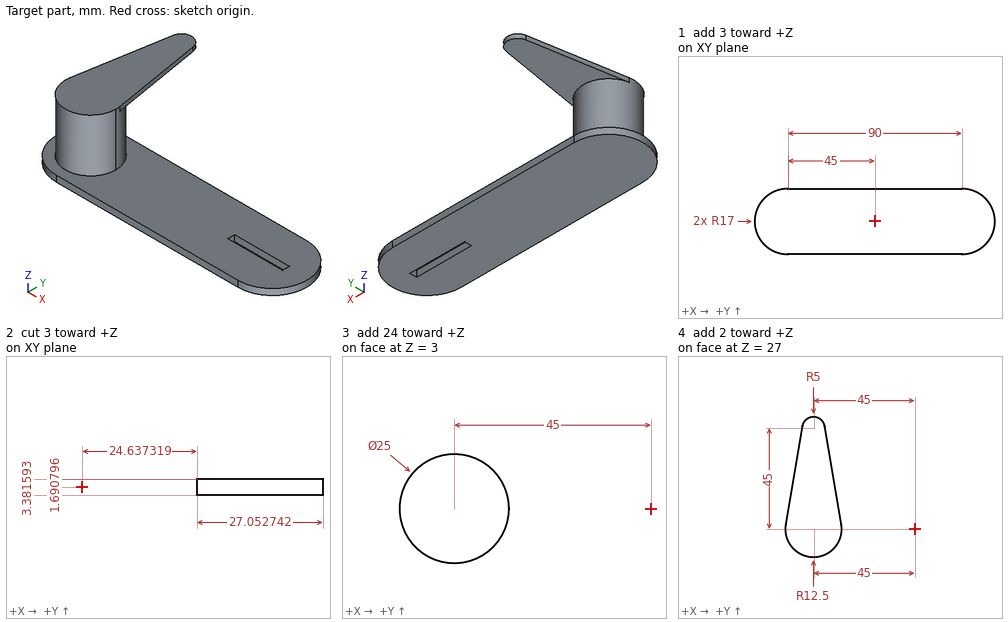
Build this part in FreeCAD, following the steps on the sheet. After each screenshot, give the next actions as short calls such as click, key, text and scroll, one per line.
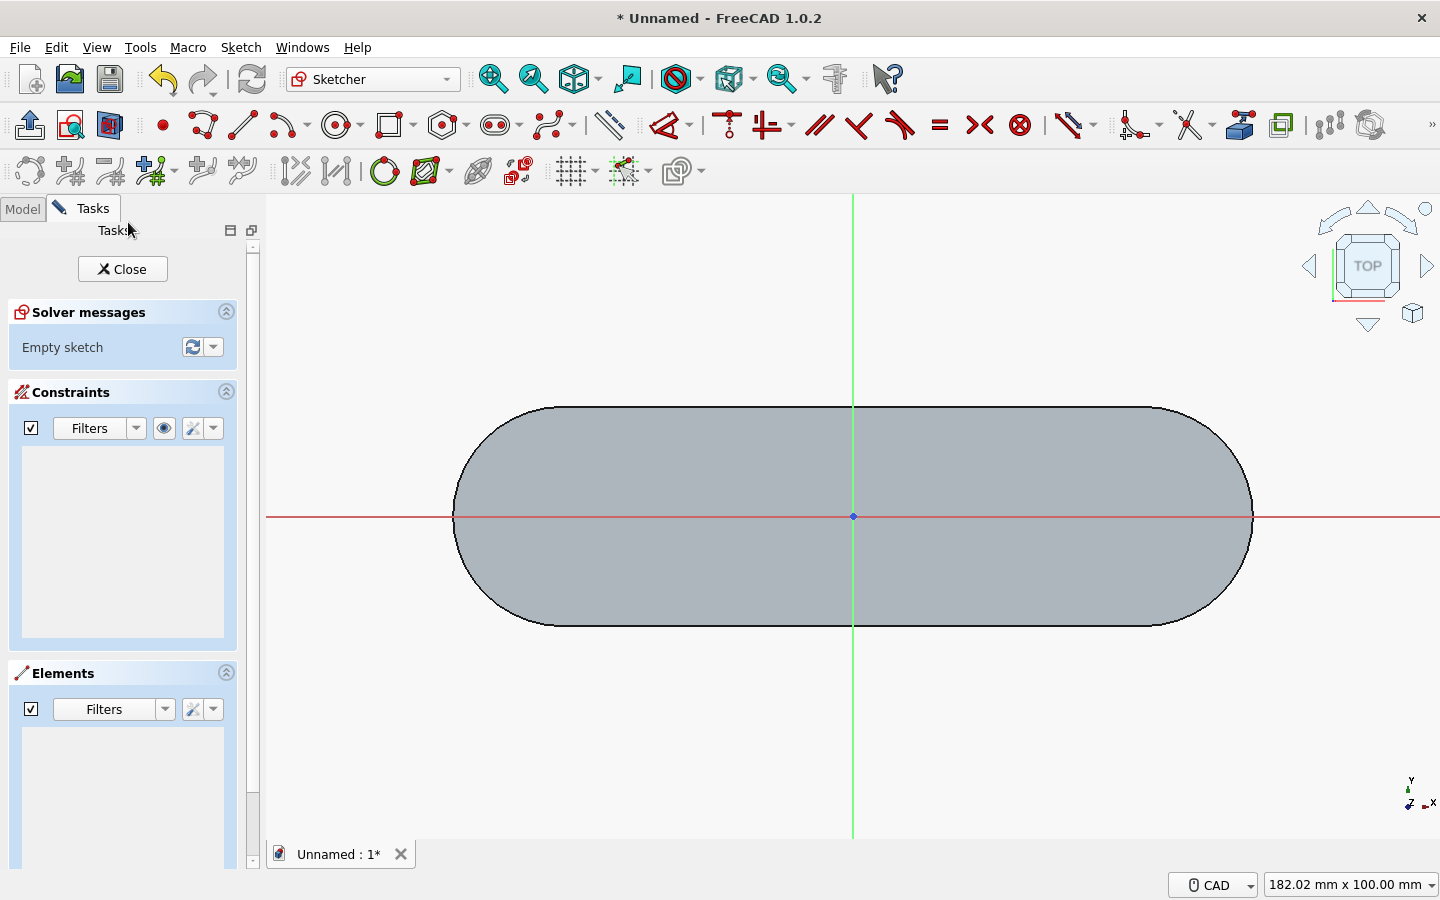
scroll(1212, 517, up, 4)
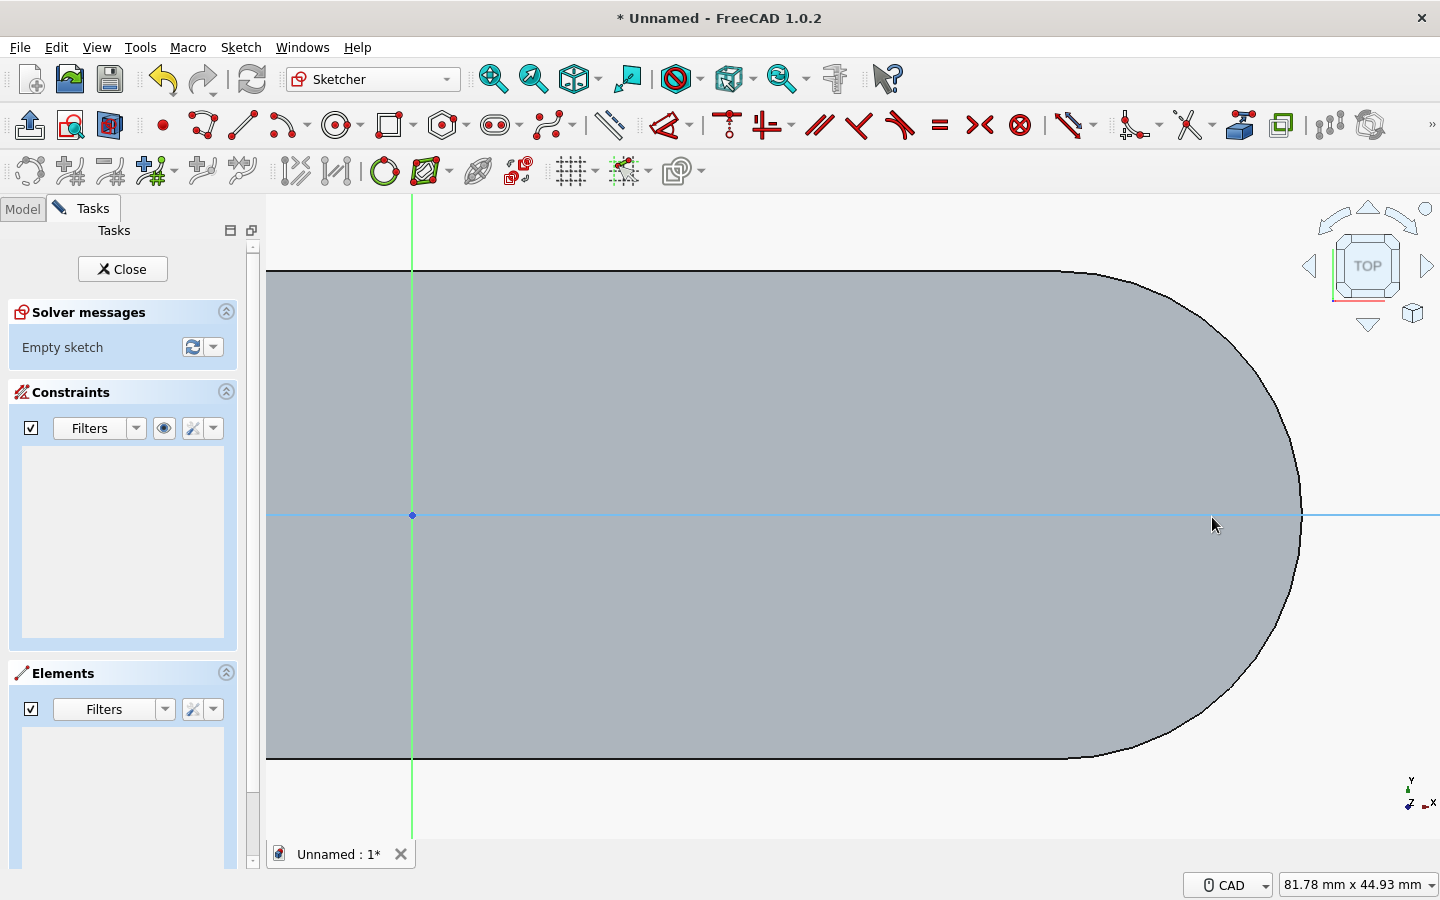
click(390, 126)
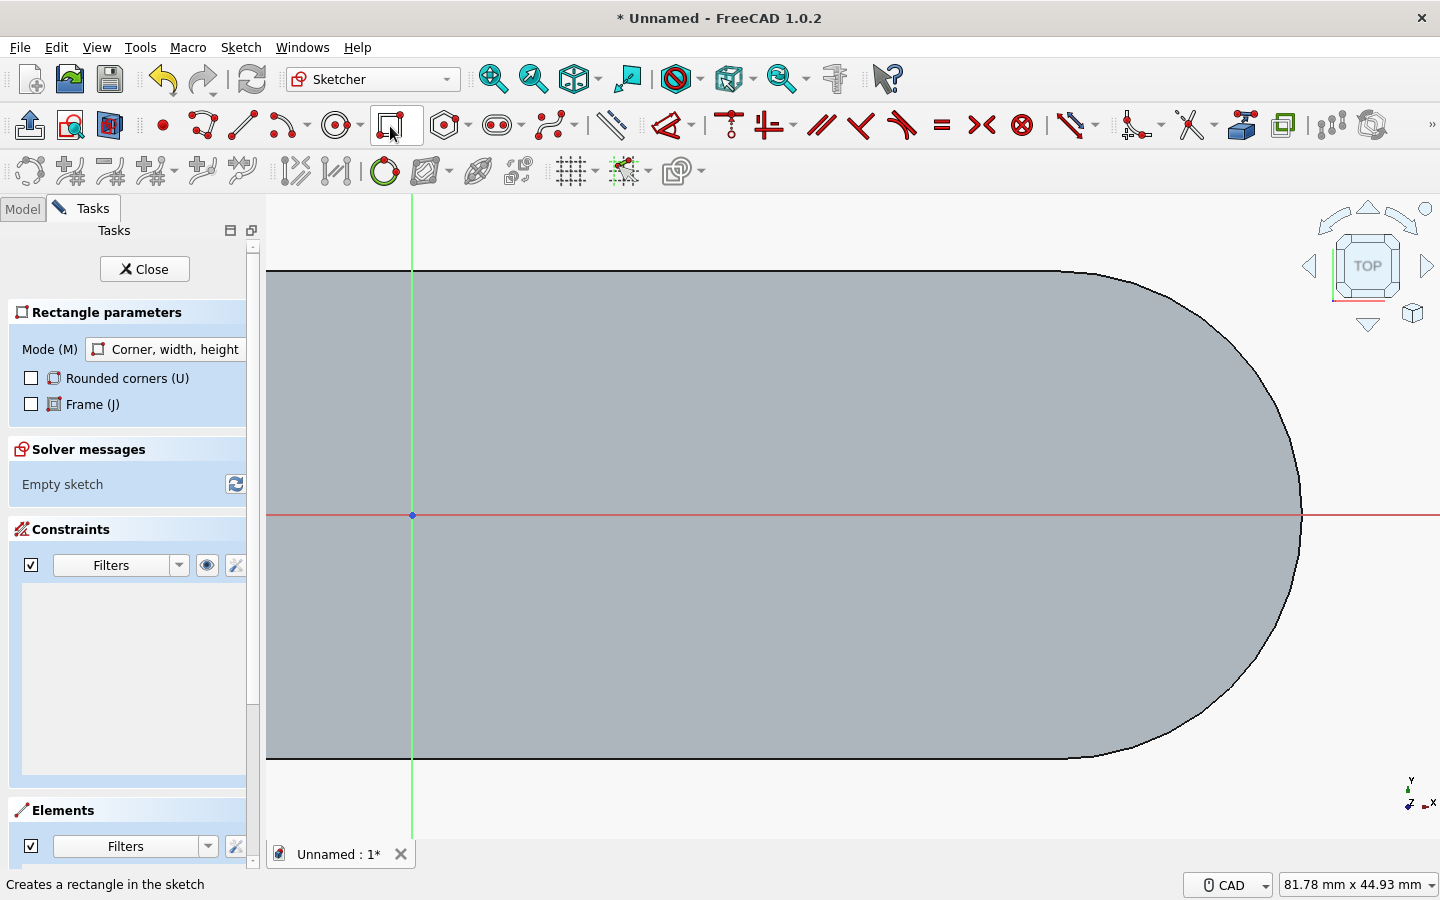
click(766, 491)
click(1154, 540)
key(Escape)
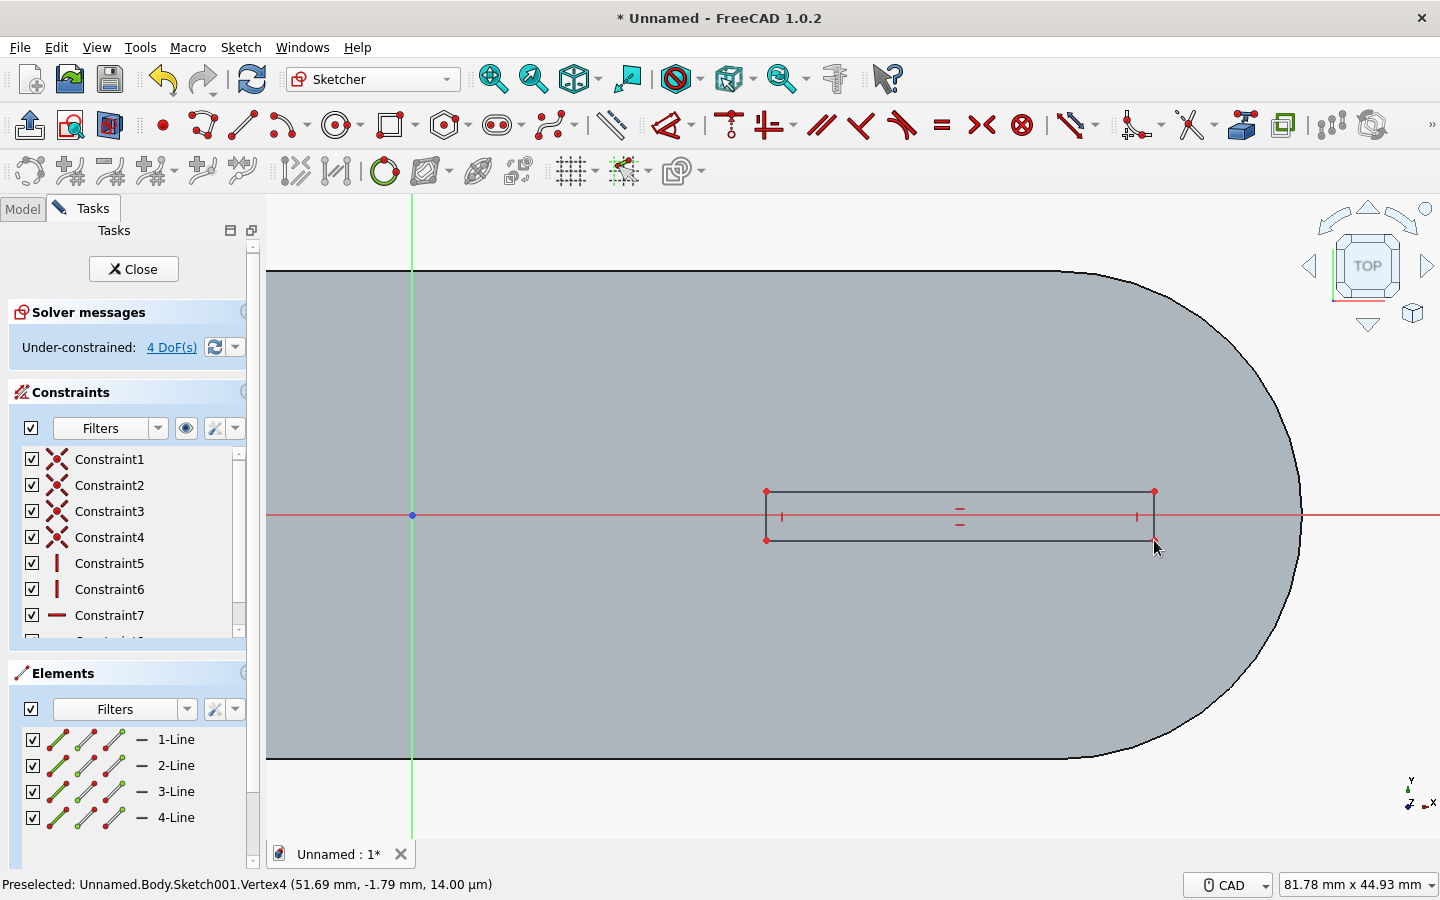
key(d)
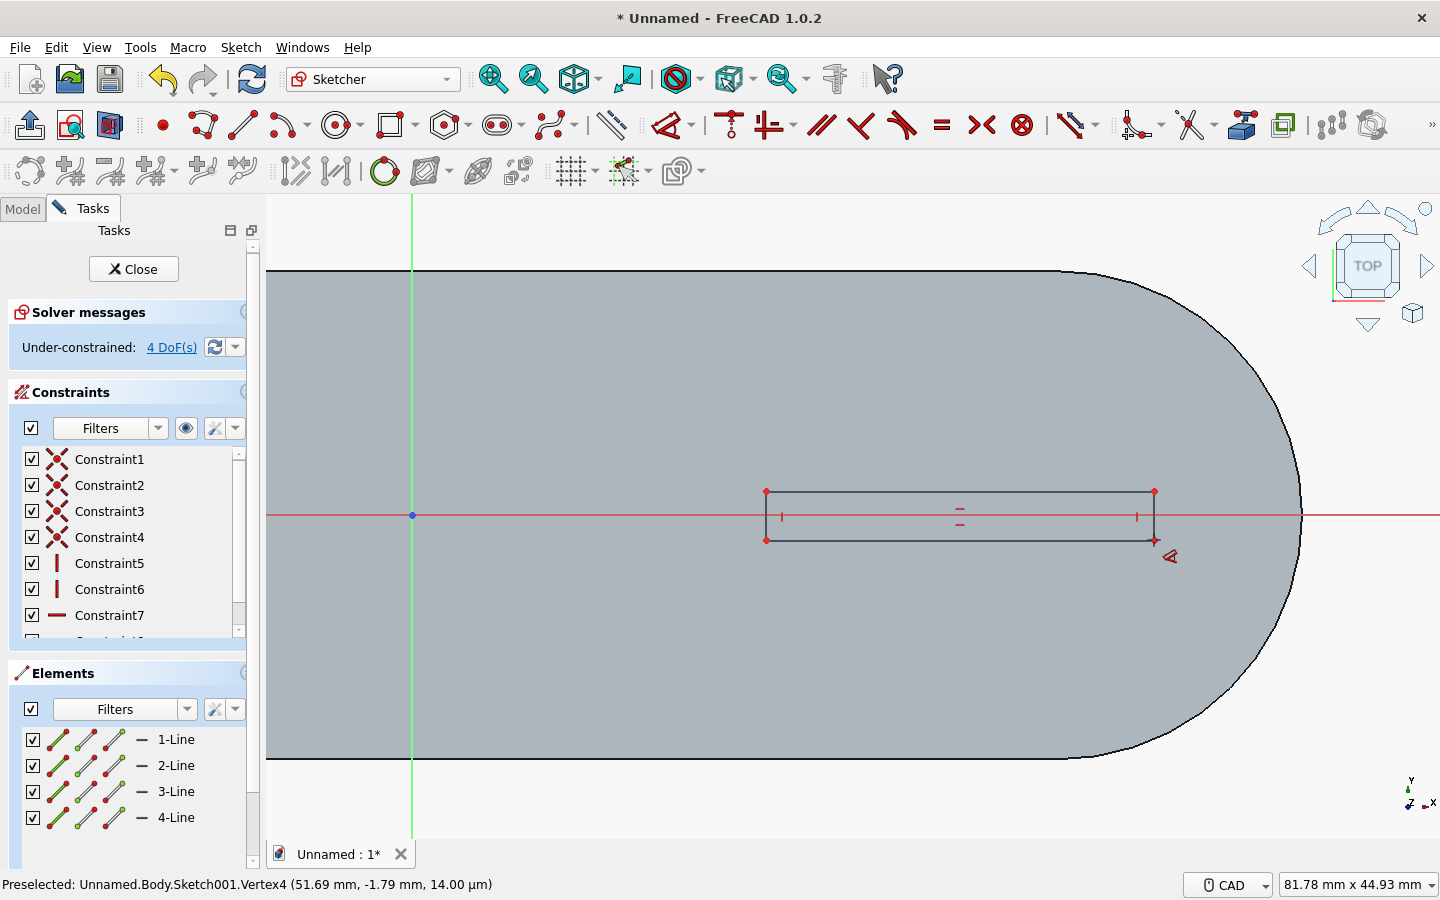
scroll(766, 526, up, 2)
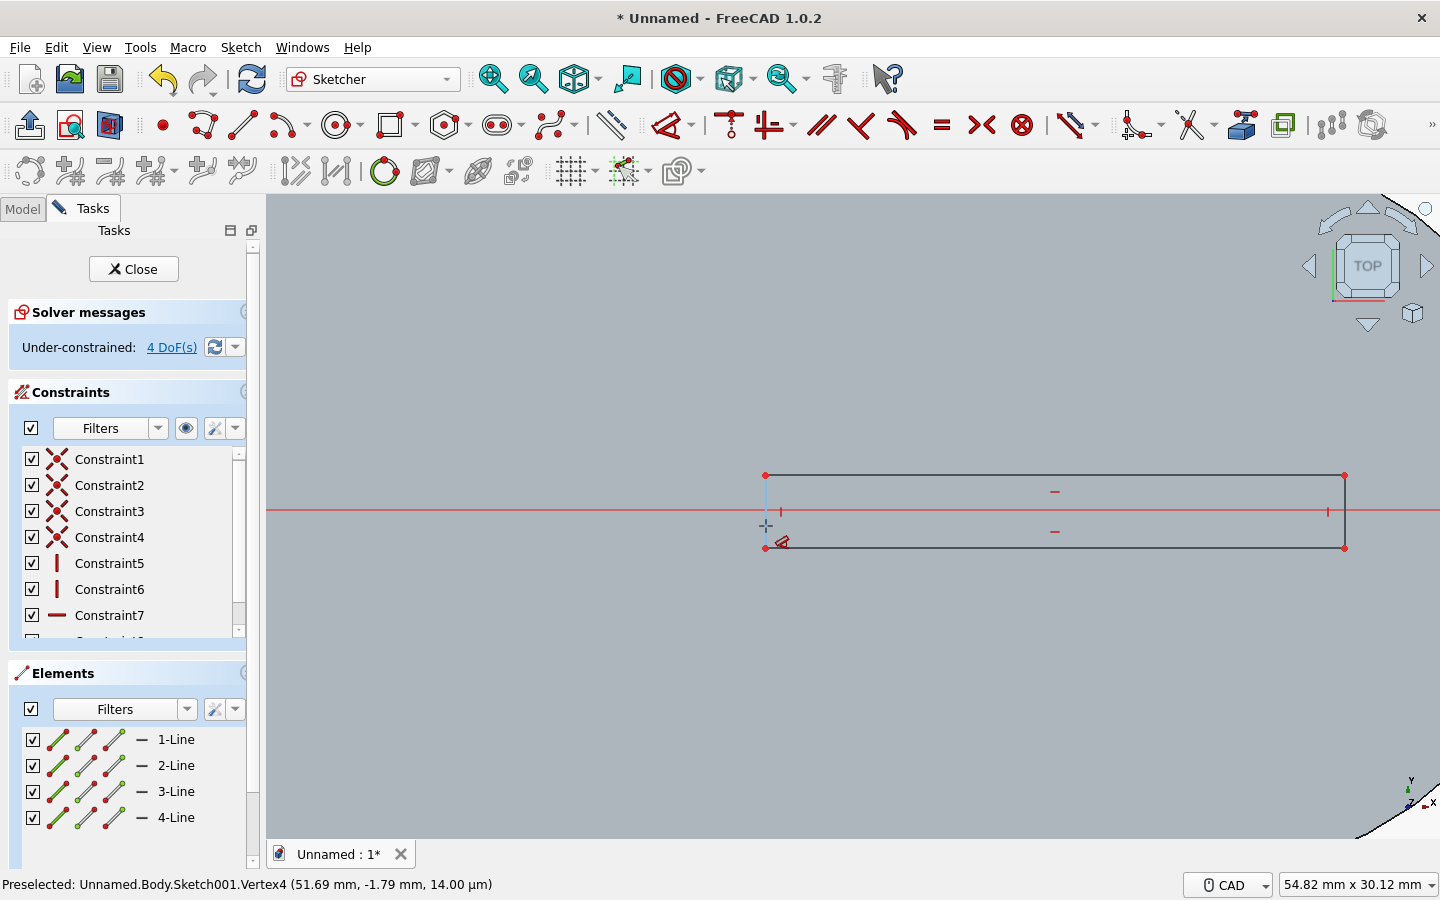
click(766, 526)
click(732, 495)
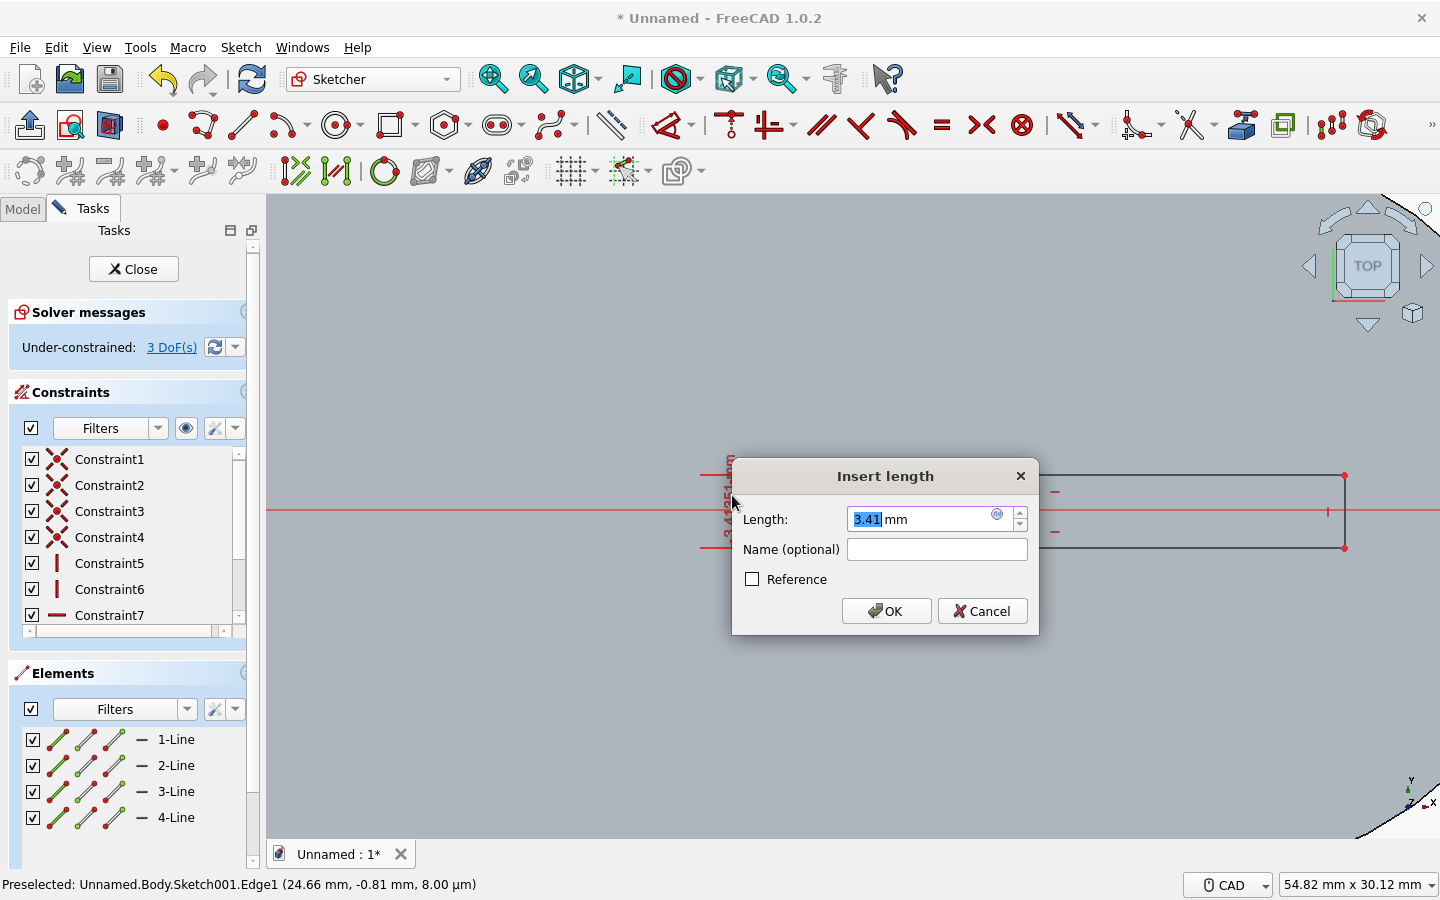
text(3.381593)
key(Return)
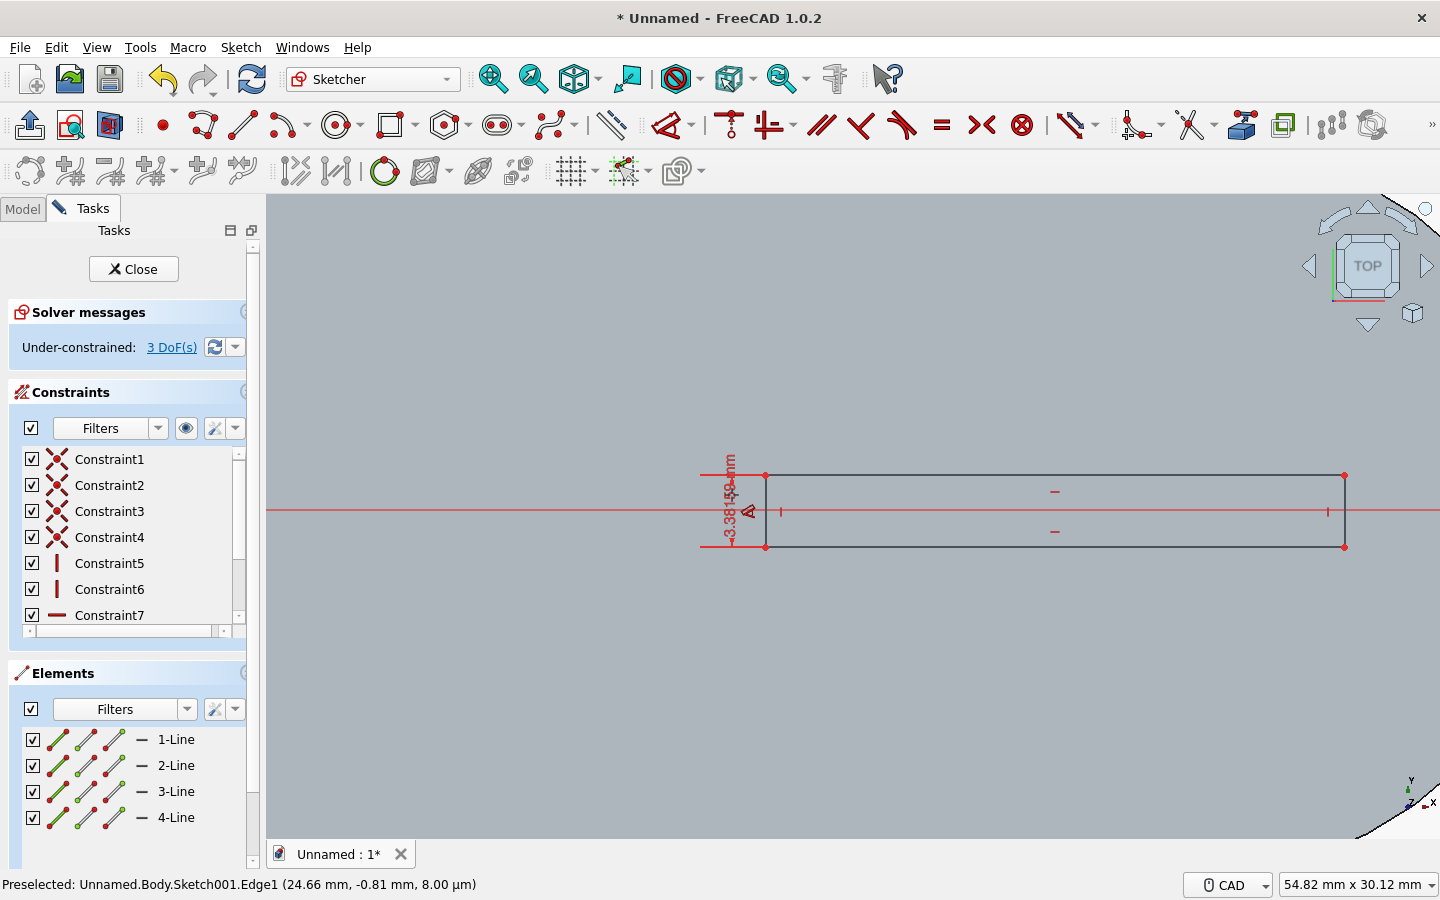
click(939, 547)
click(1020, 581)